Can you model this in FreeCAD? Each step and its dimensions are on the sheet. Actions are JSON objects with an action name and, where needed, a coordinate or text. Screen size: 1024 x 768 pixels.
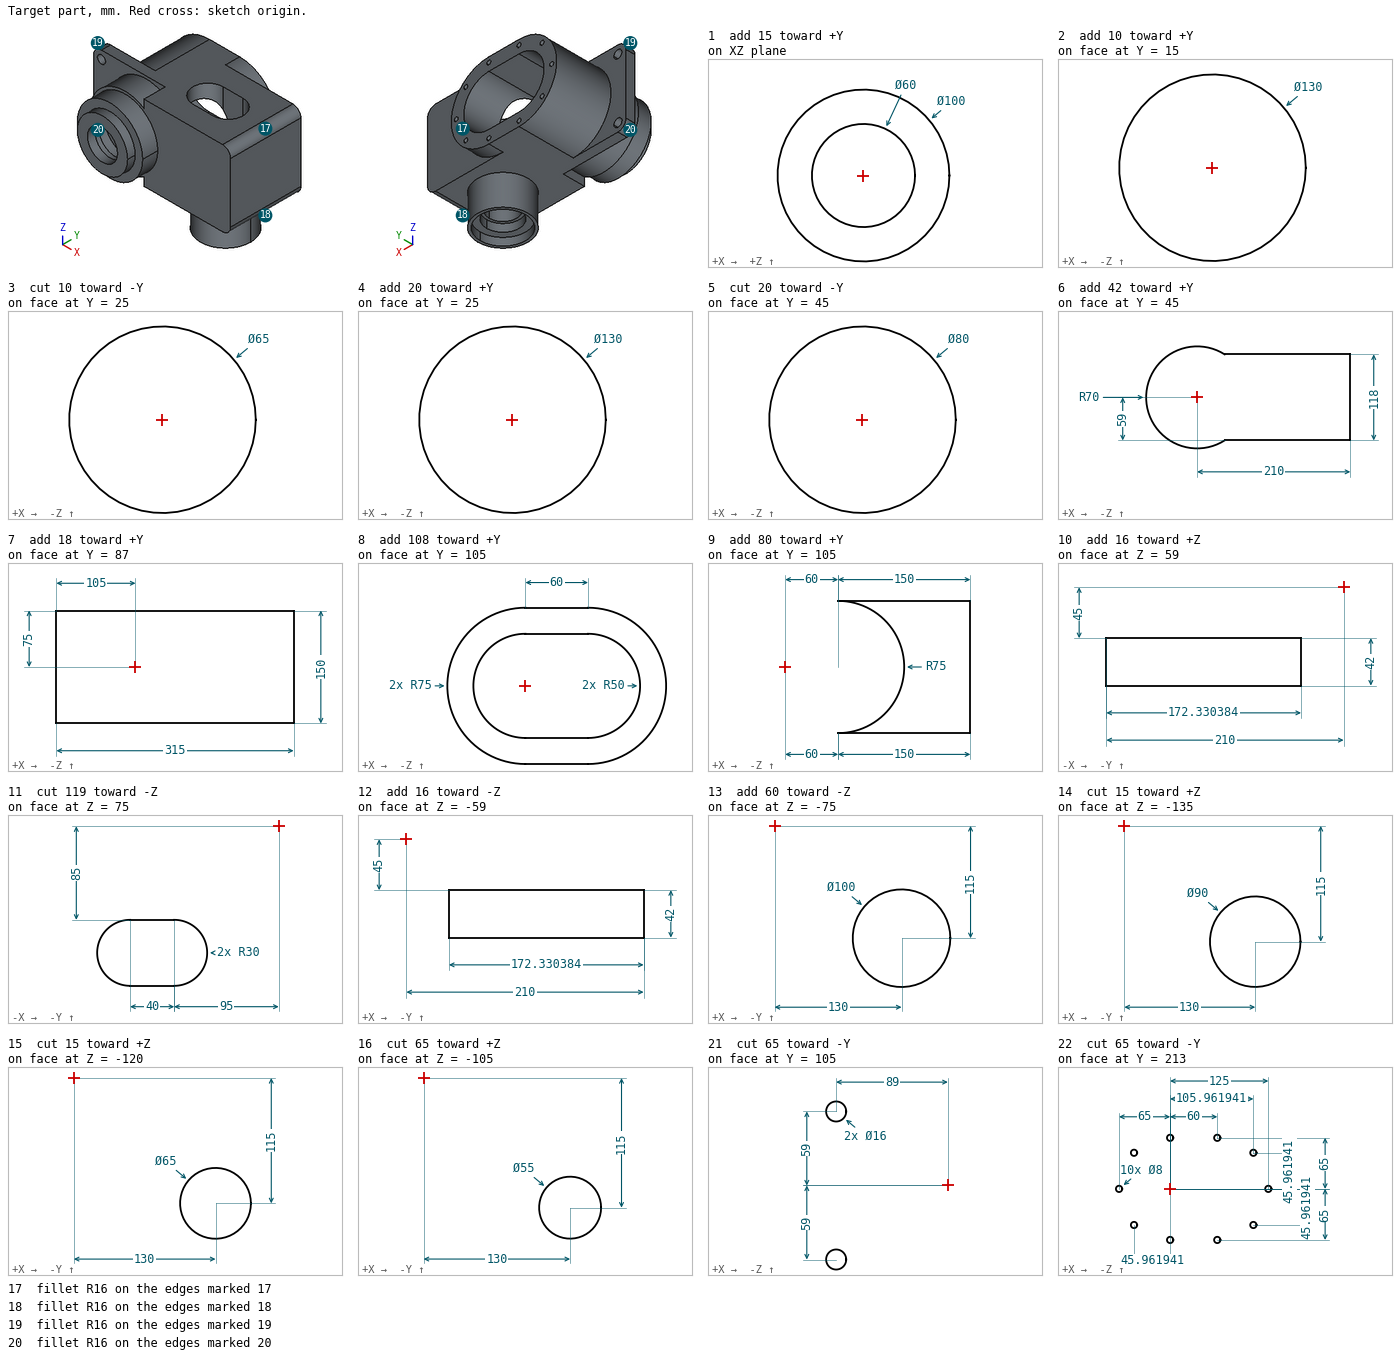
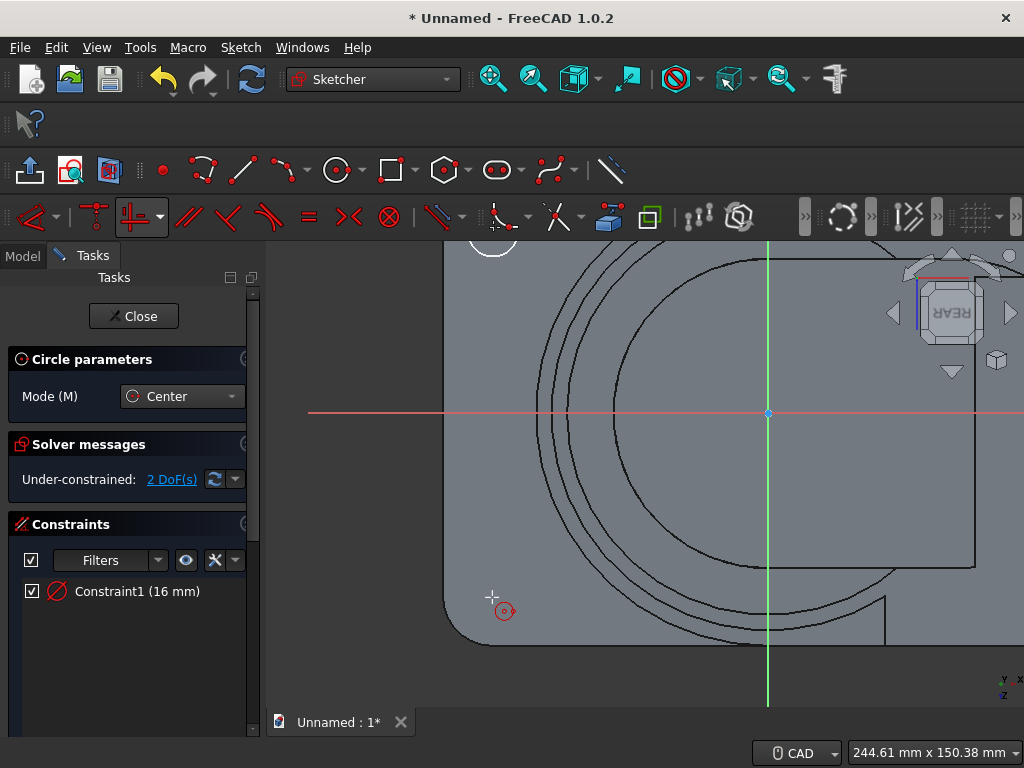
{"action": "left_click", "coordinate": [493, 596]}
{"action": "mouse_move", "coordinate": [510, 579]}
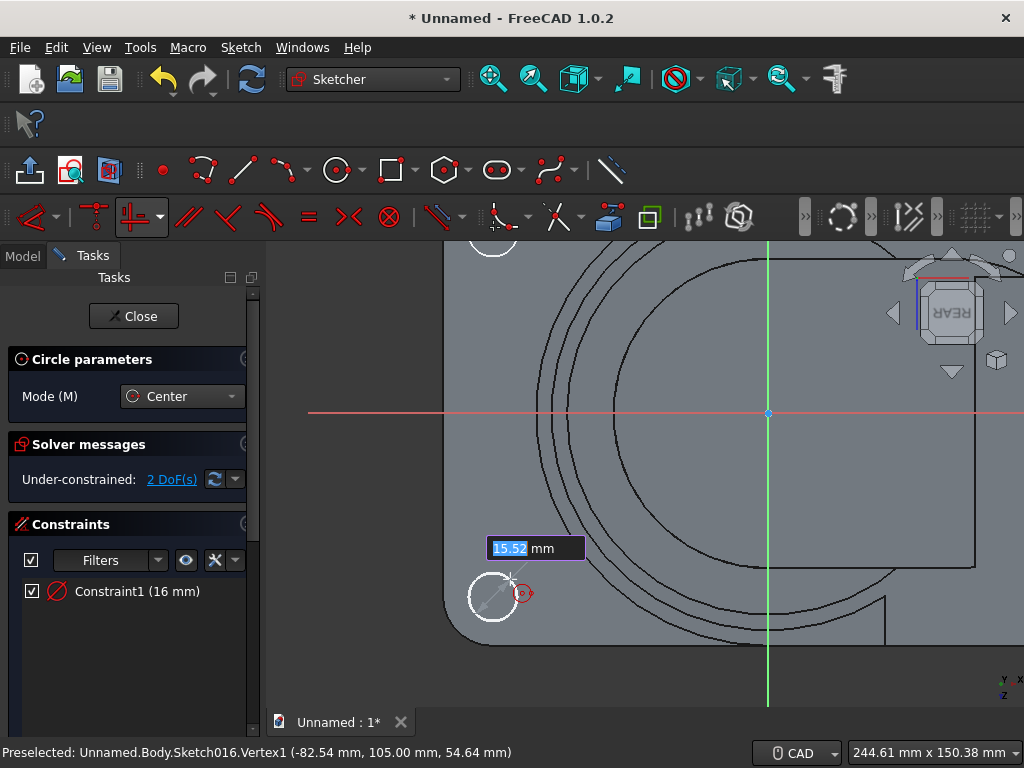
{"action": "type", "text": "16"}
{"action": "key", "text": "Return"}
{"action": "key", "text": "Escape"}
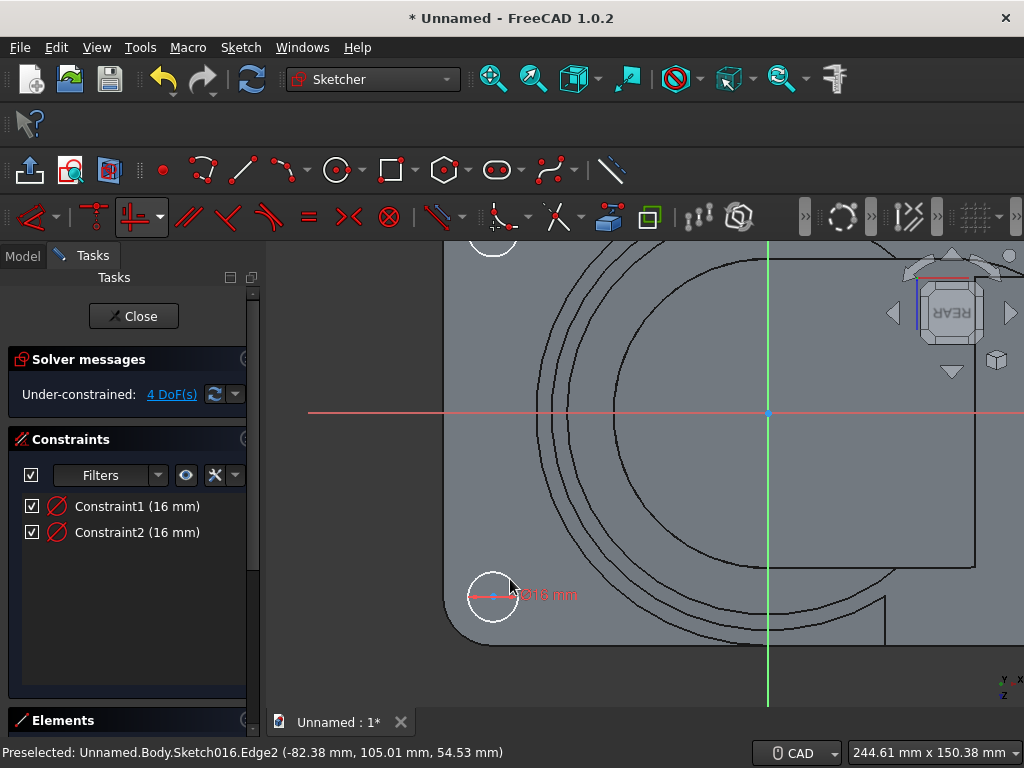
{"action": "scroll", "coordinate": [492, 597], "scroll_direction": "down", "scroll_amount": 2}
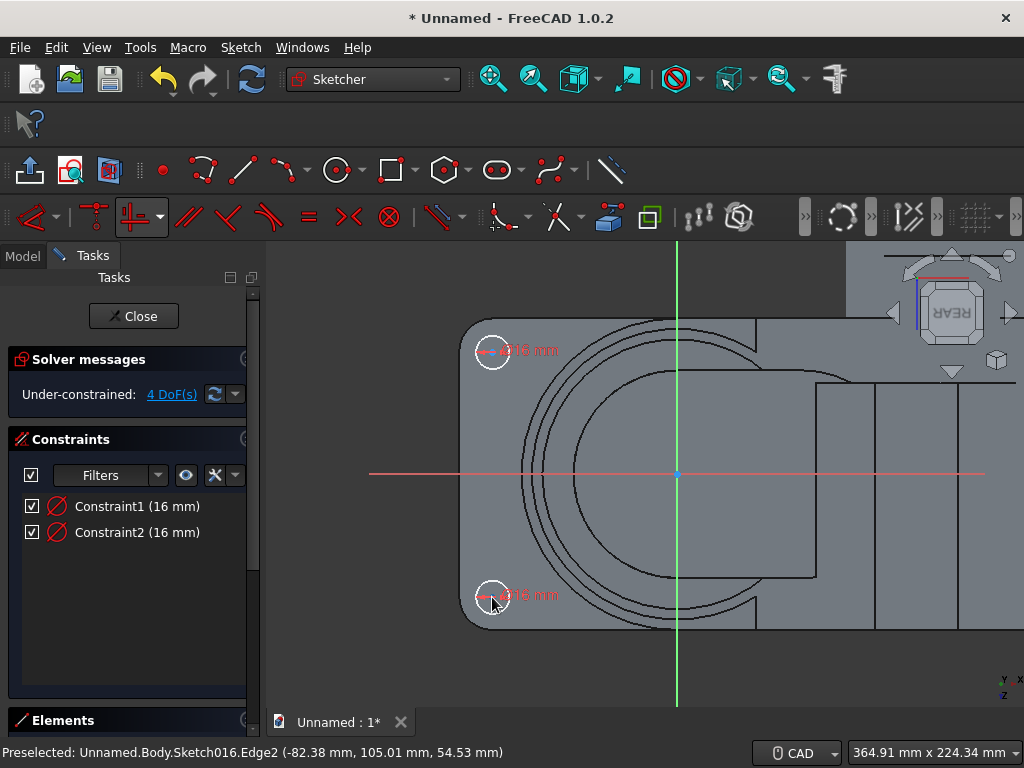
{"action": "left_click", "coordinate": [493, 352]}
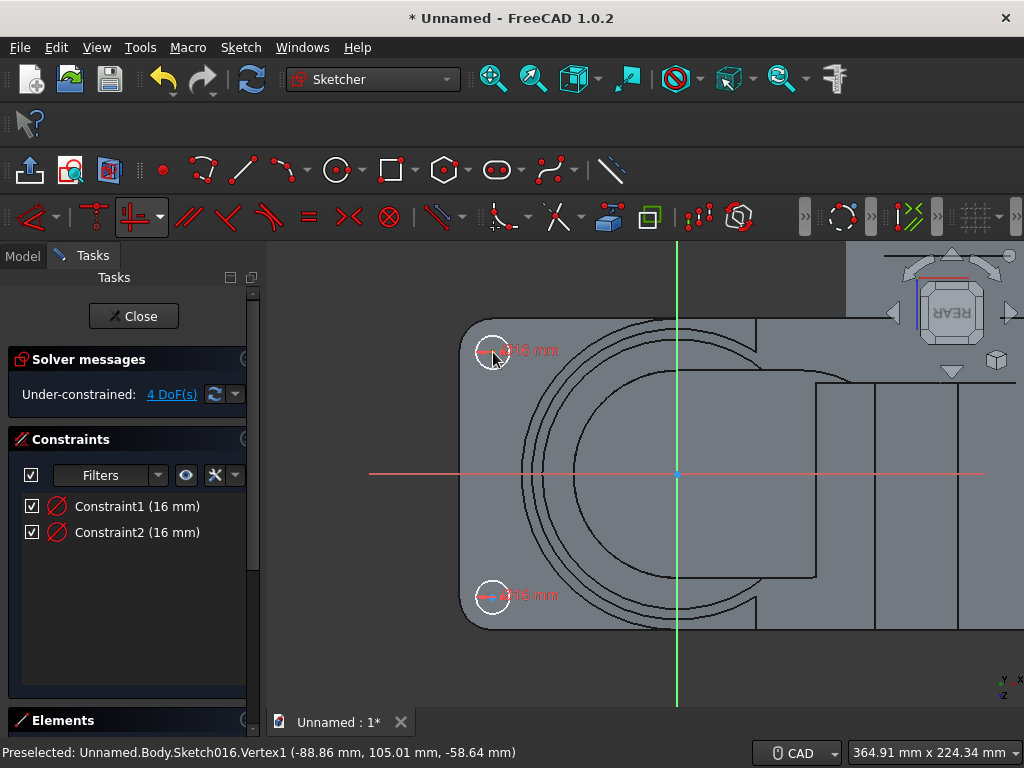
{"action": "left_click", "coordinate": [493, 597]}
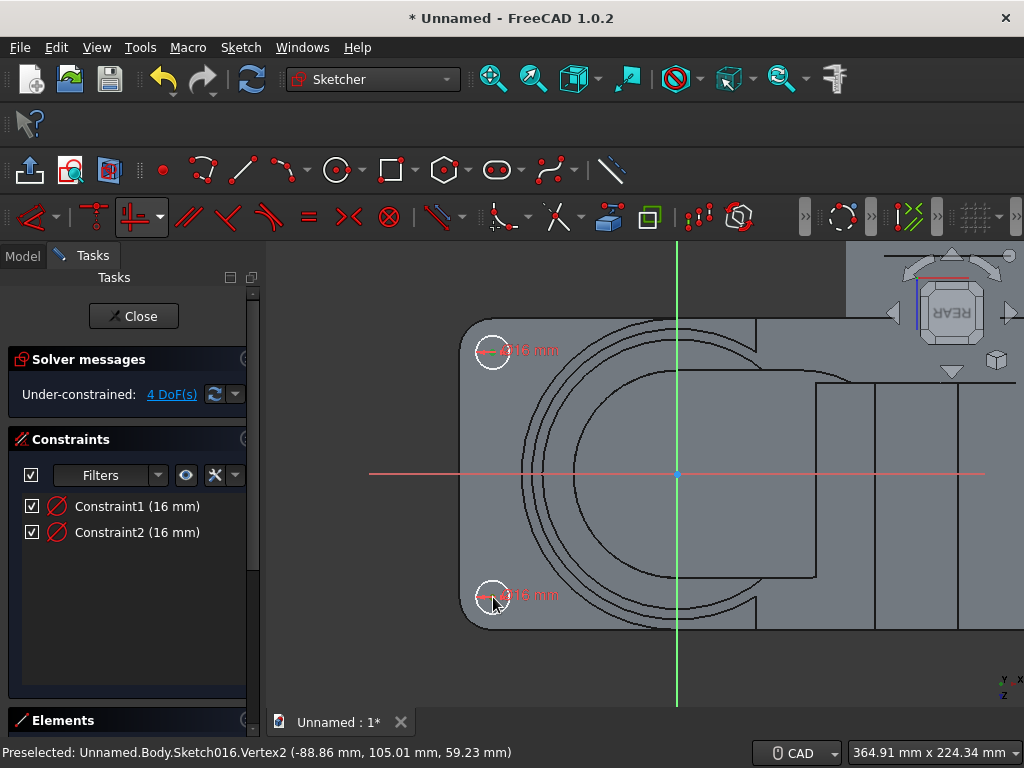
{"action": "left_click", "coordinate": [162, 218]}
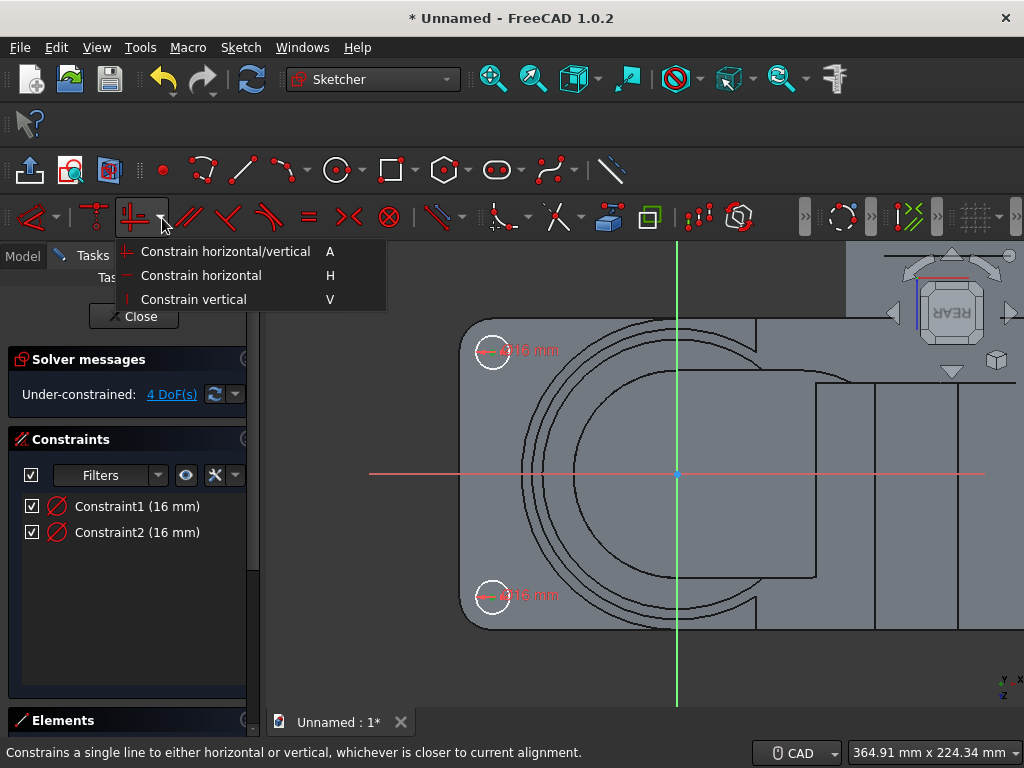
{"action": "left_click", "coordinate": [251, 299]}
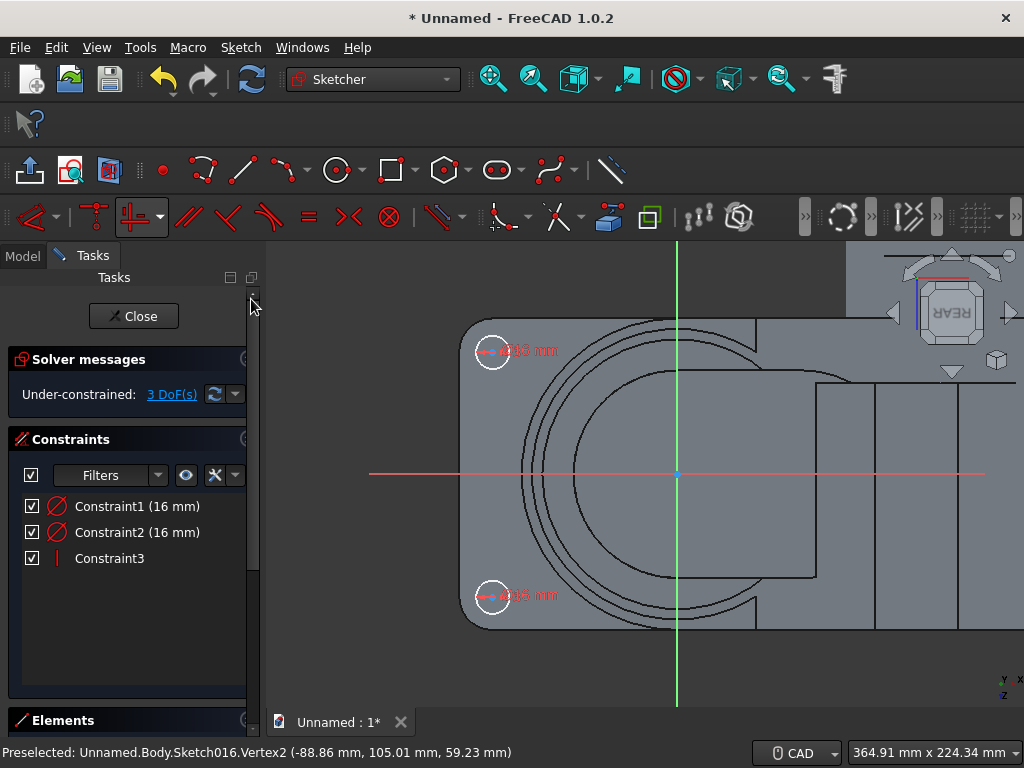
{"action": "left_click", "coordinate": [32, 218]}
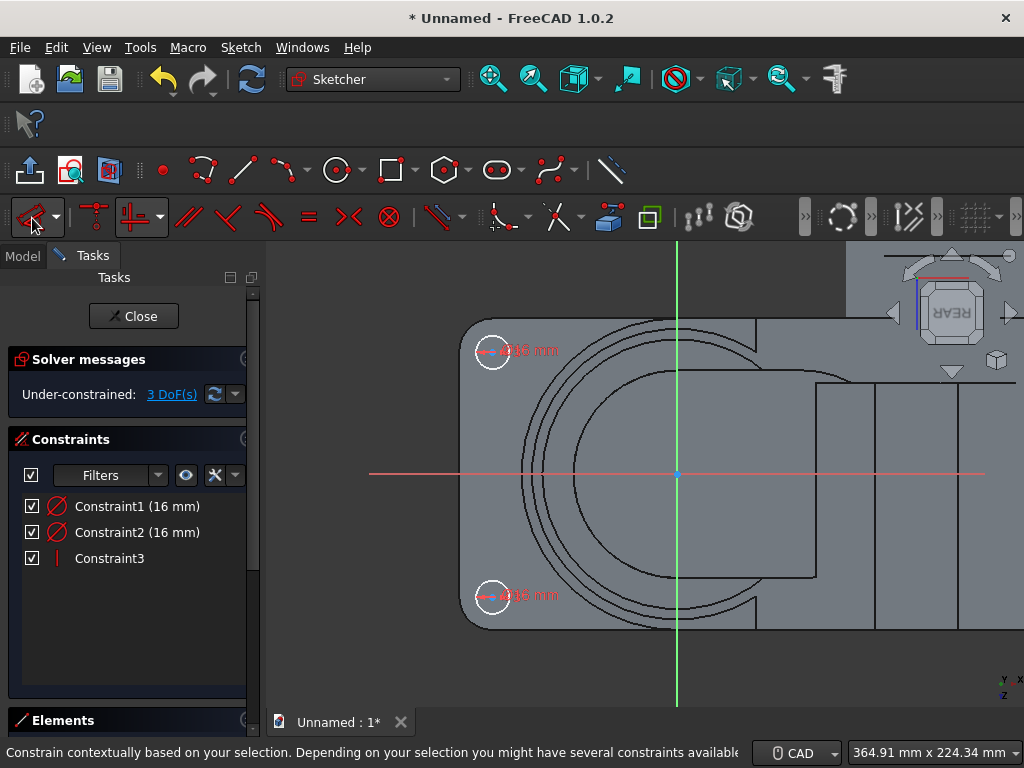
{"action": "left_click", "coordinate": [493, 352]}
{"action": "left_click", "coordinate": [585, 318]}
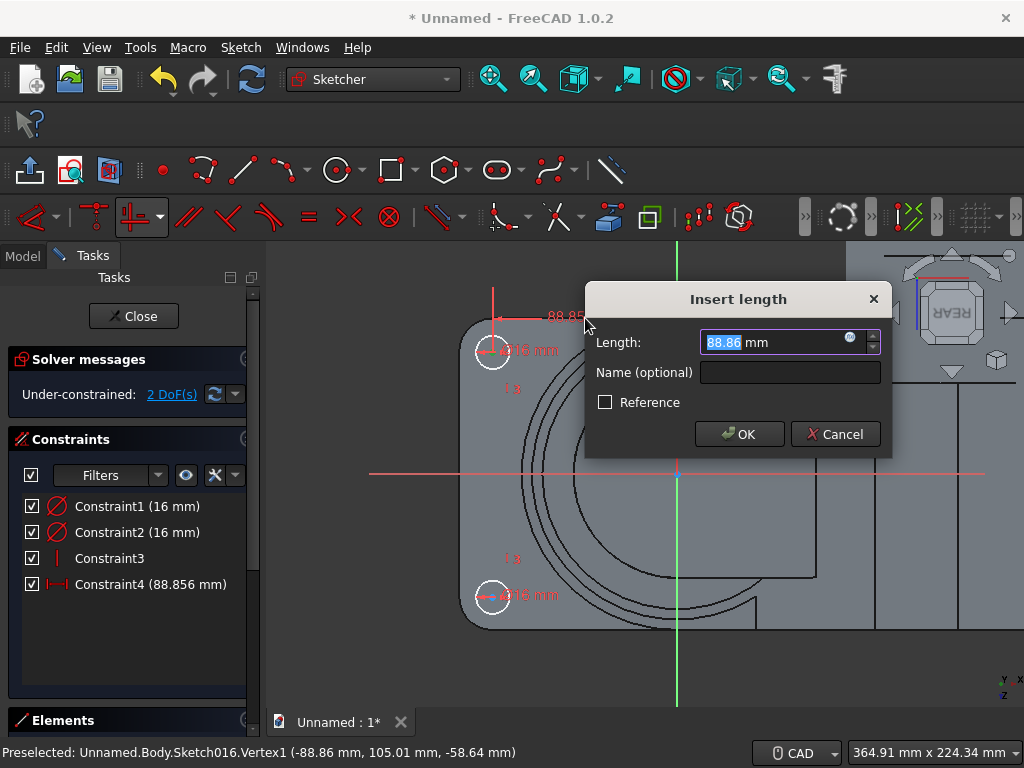
{"action": "type", "text": "89"}
{"action": "key", "text": "Return"}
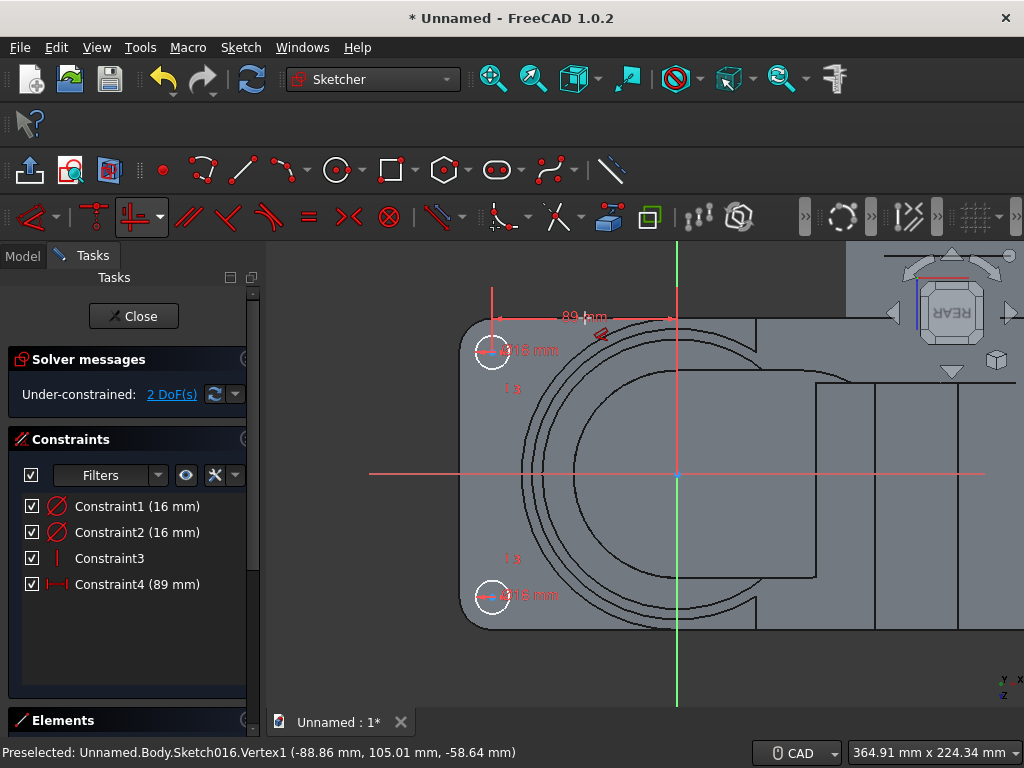
{"action": "left_click", "coordinate": [492, 352]}
{"action": "left_click", "coordinate": [711, 413]}